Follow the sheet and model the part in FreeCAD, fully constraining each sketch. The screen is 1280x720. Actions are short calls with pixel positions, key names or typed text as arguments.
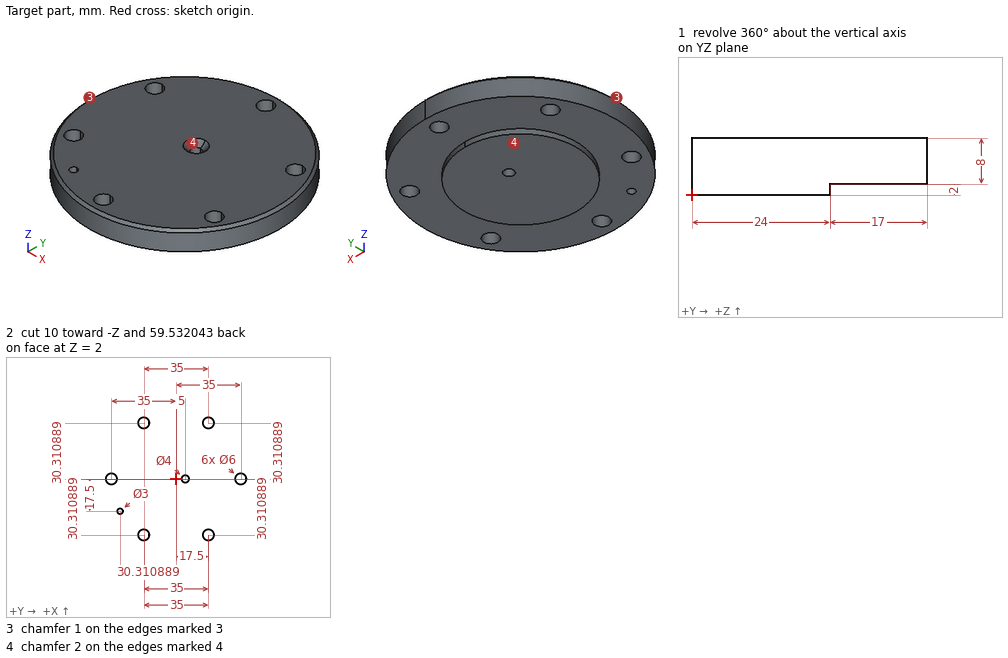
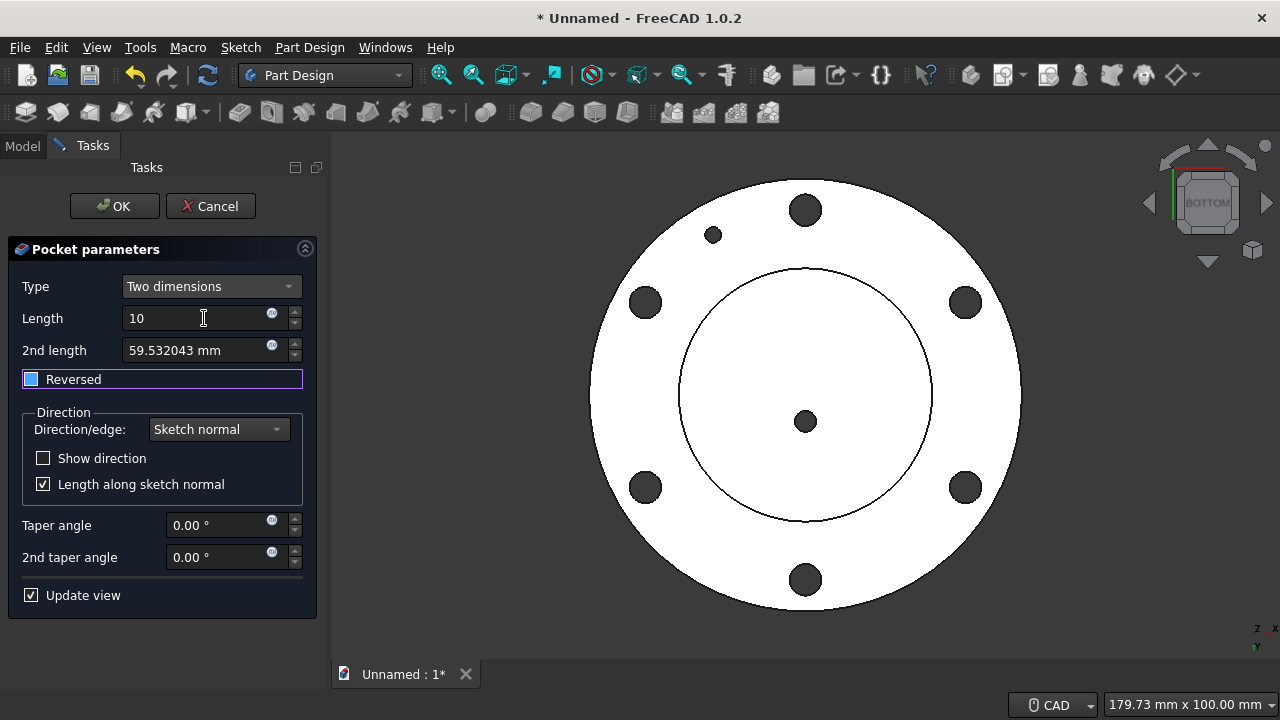
click(30, 379)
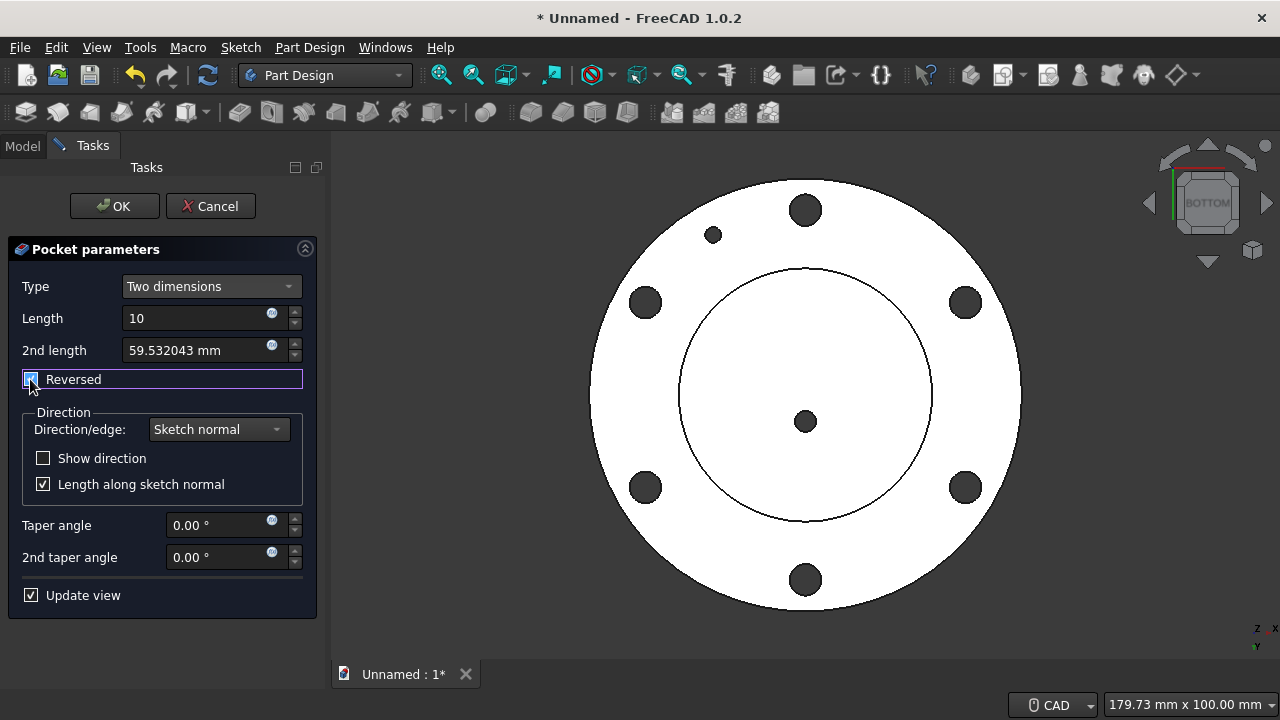
click(115, 206)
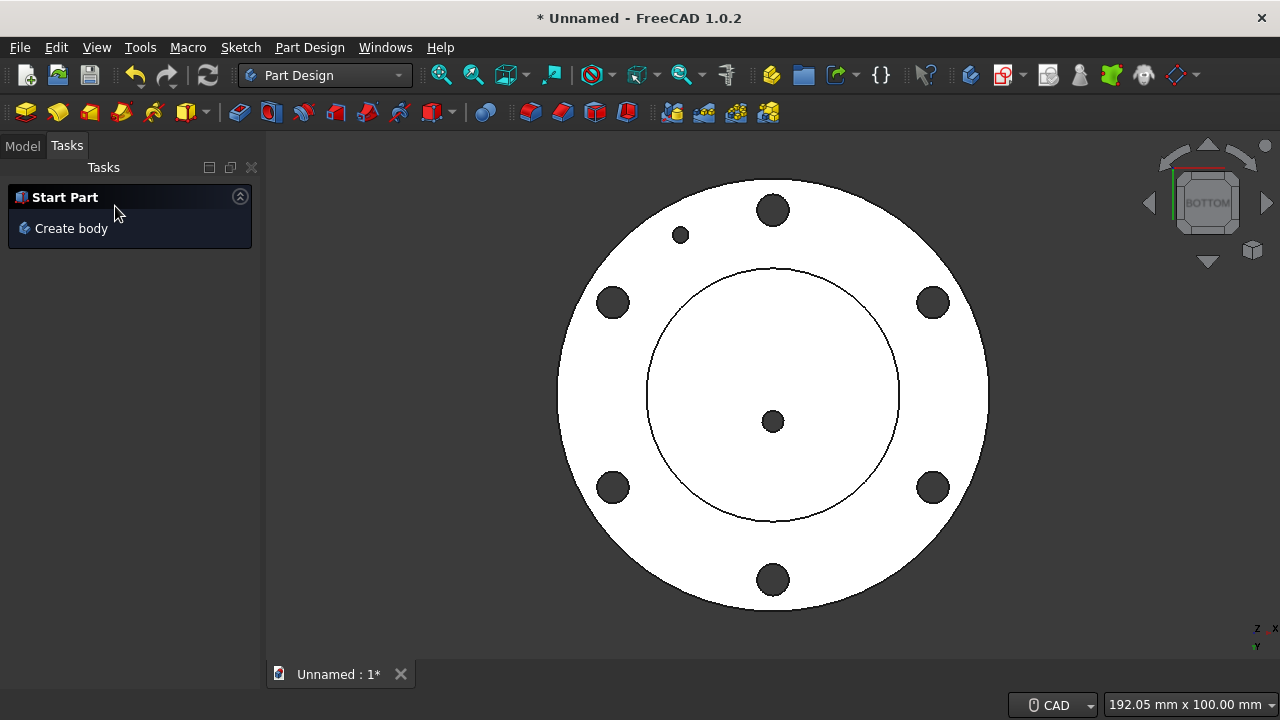
key(0)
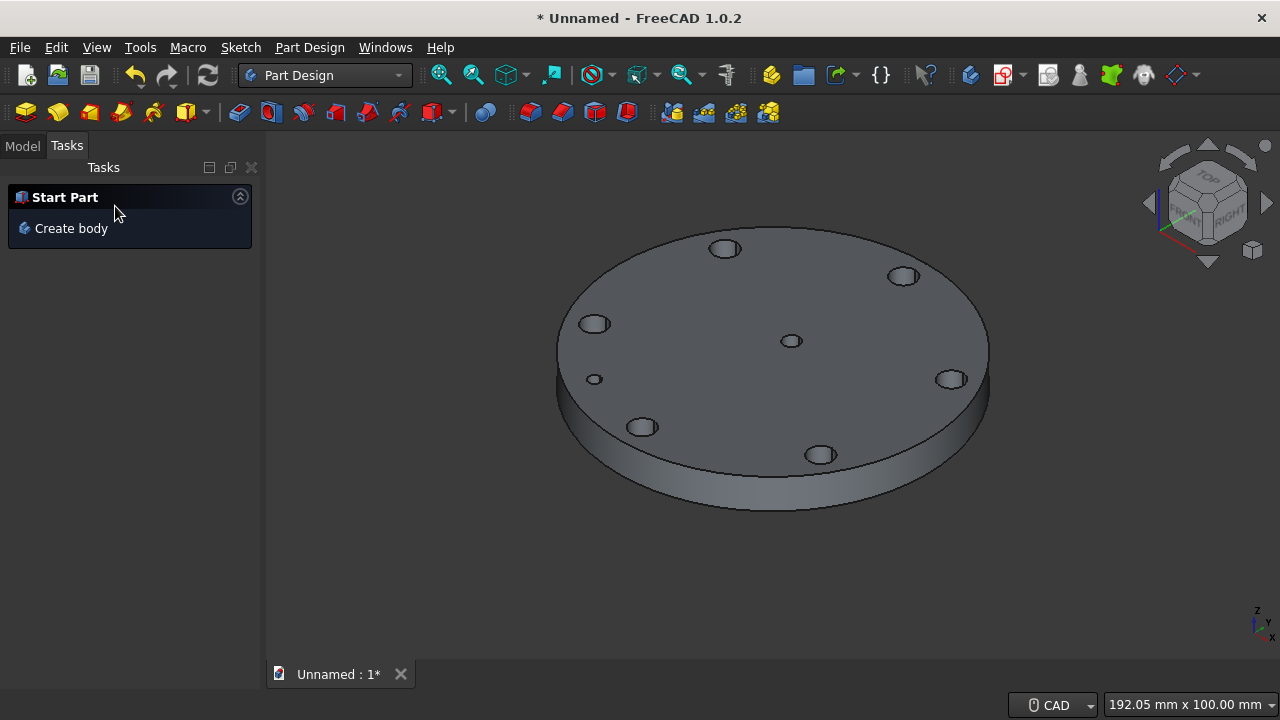
click(620, 439)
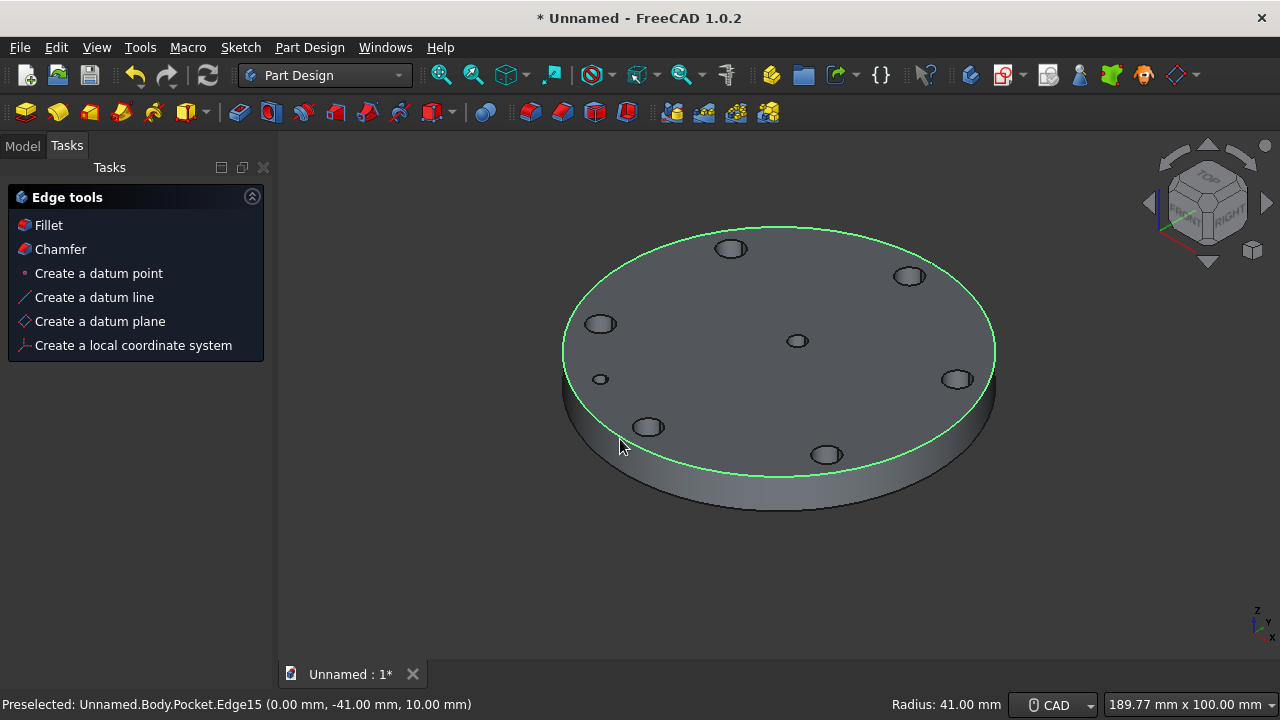
click(564, 112)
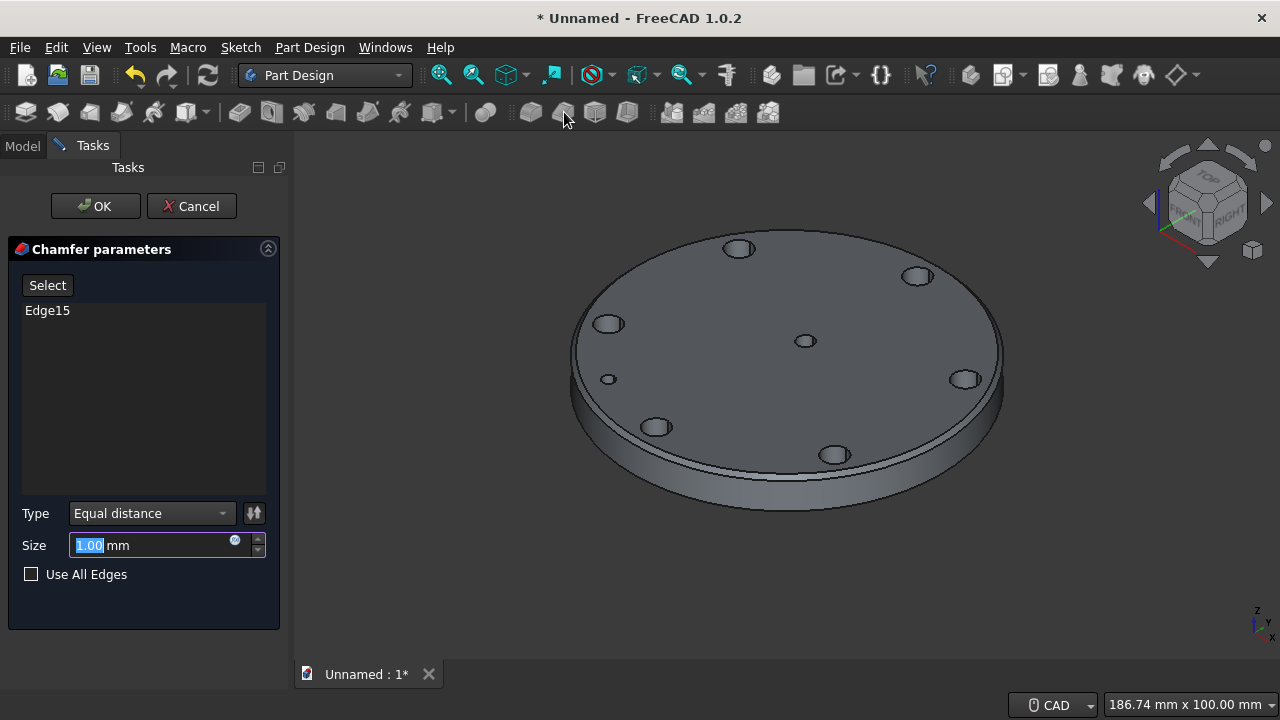
text(1)
key(Tab)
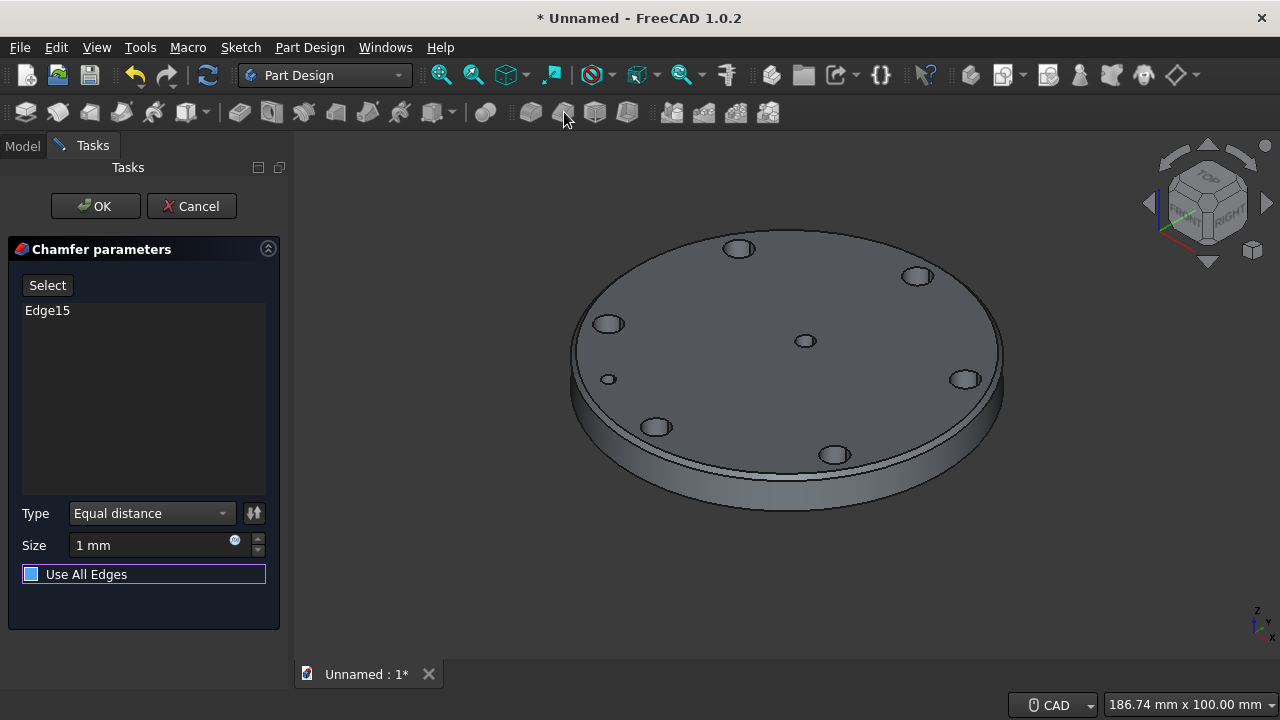
click(96, 206)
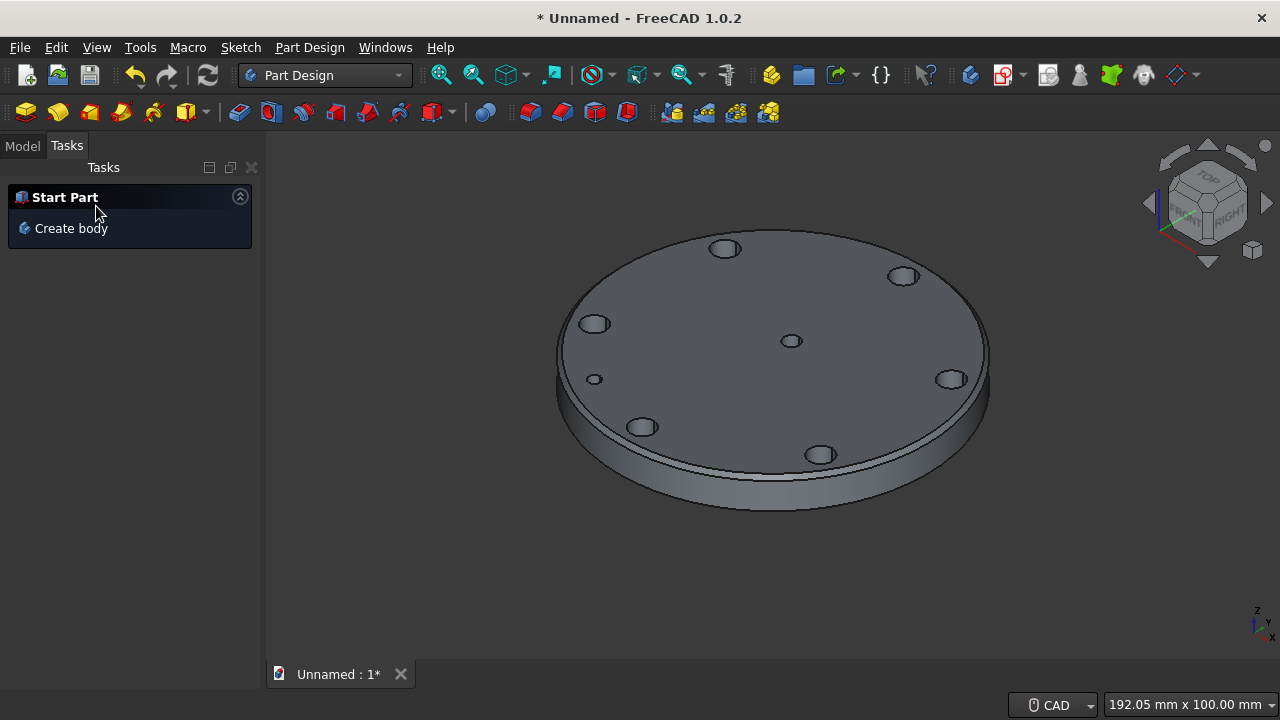
click(784, 344)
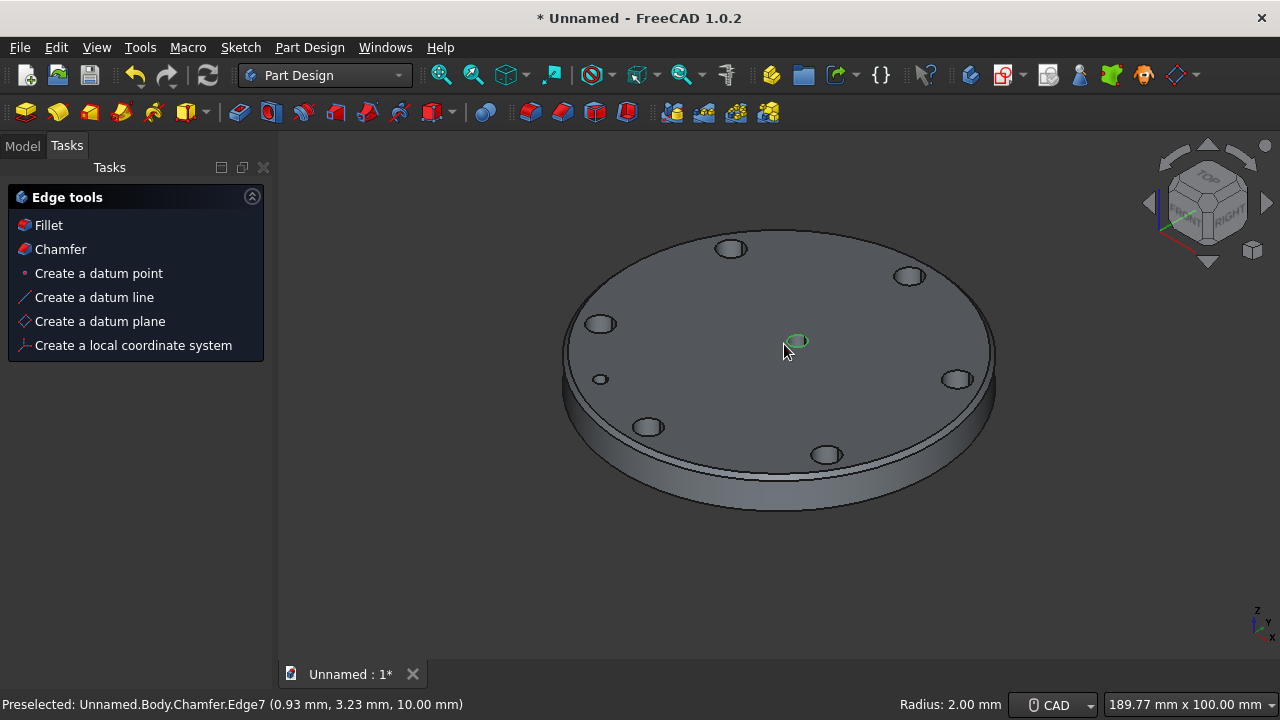
click(564, 112)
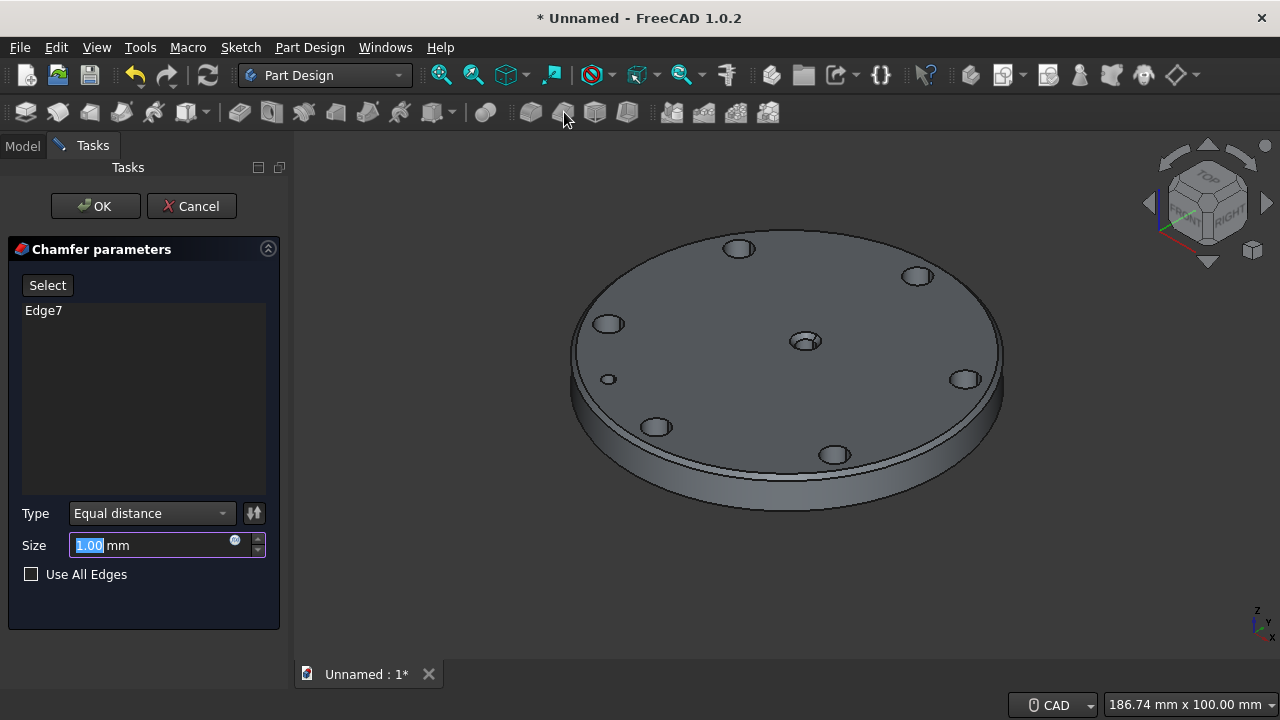
text(2)
key(Tab)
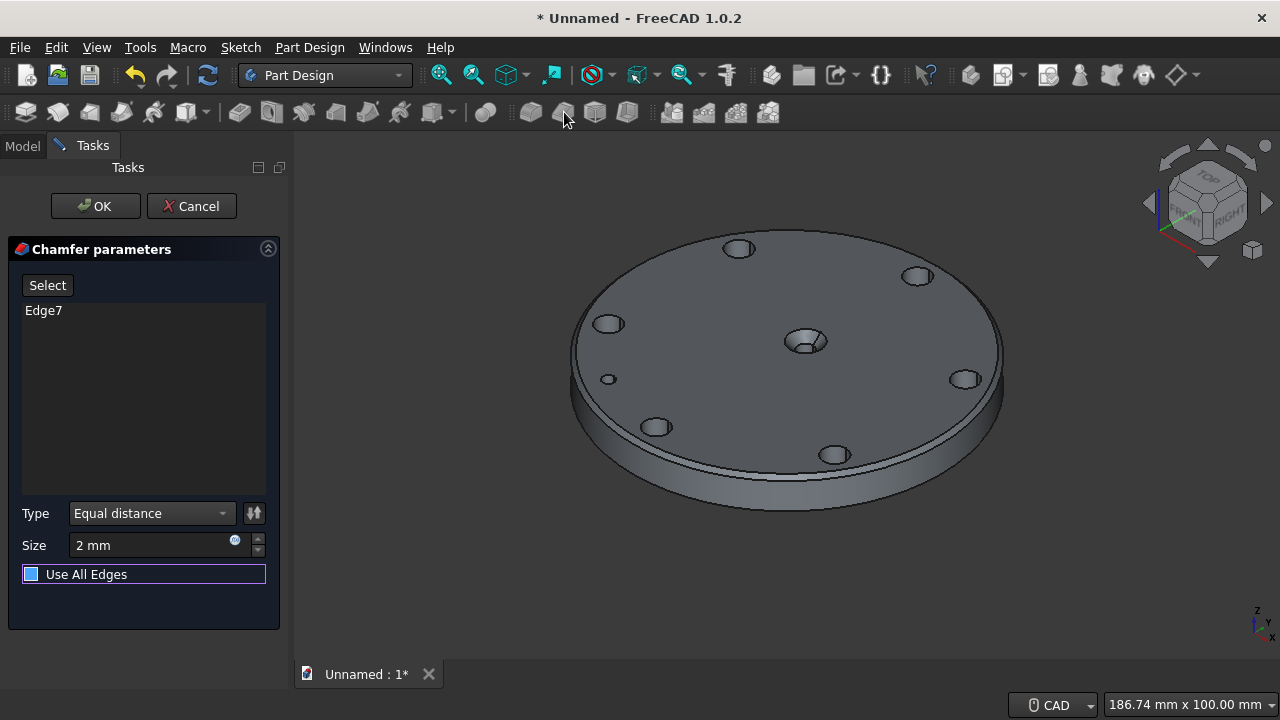
click(96, 206)